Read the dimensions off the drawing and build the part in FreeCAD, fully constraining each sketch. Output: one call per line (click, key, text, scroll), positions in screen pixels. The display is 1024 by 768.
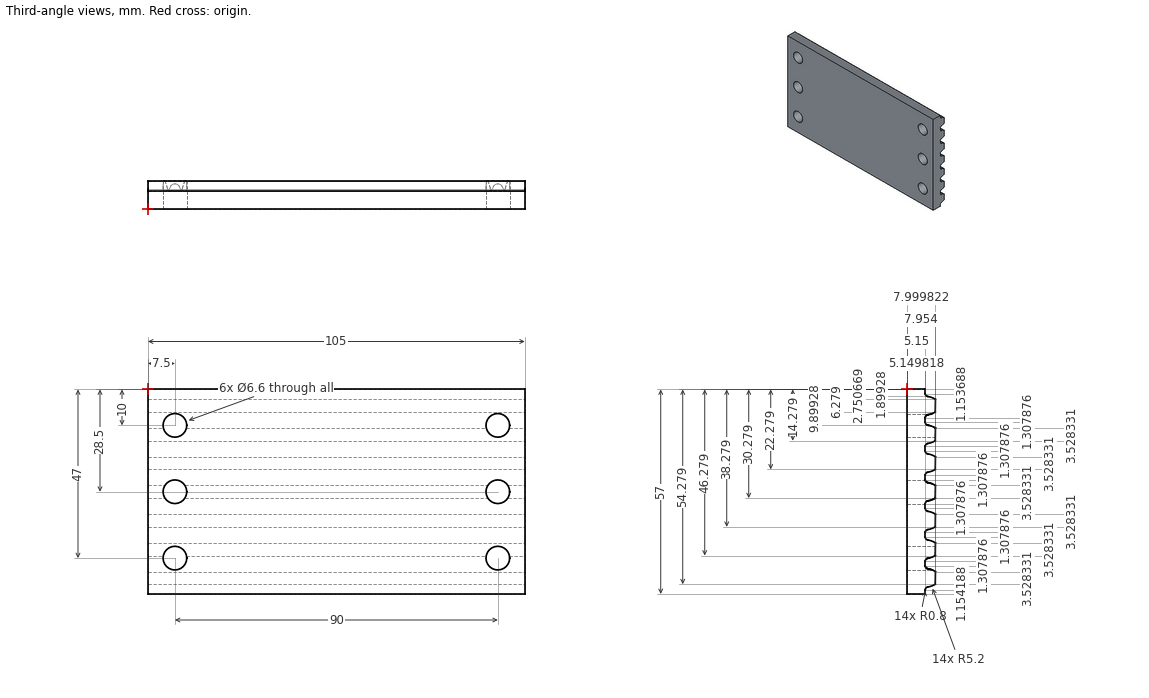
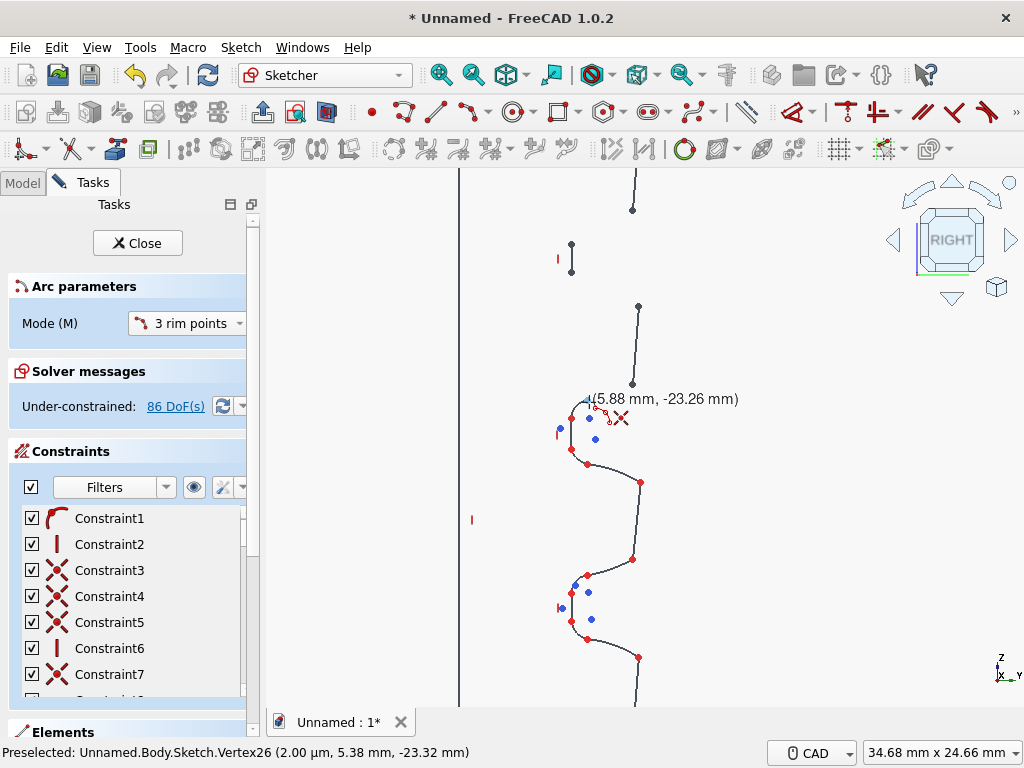
click(587, 401)
click(633, 385)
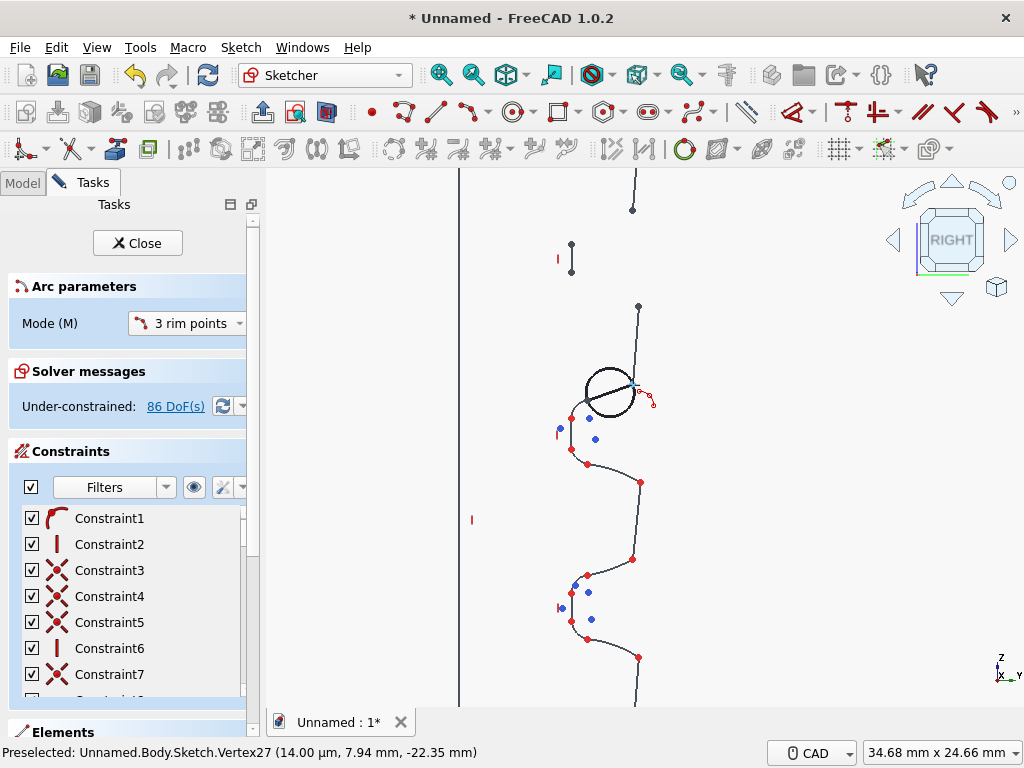
scroll(611, 394, up, 9)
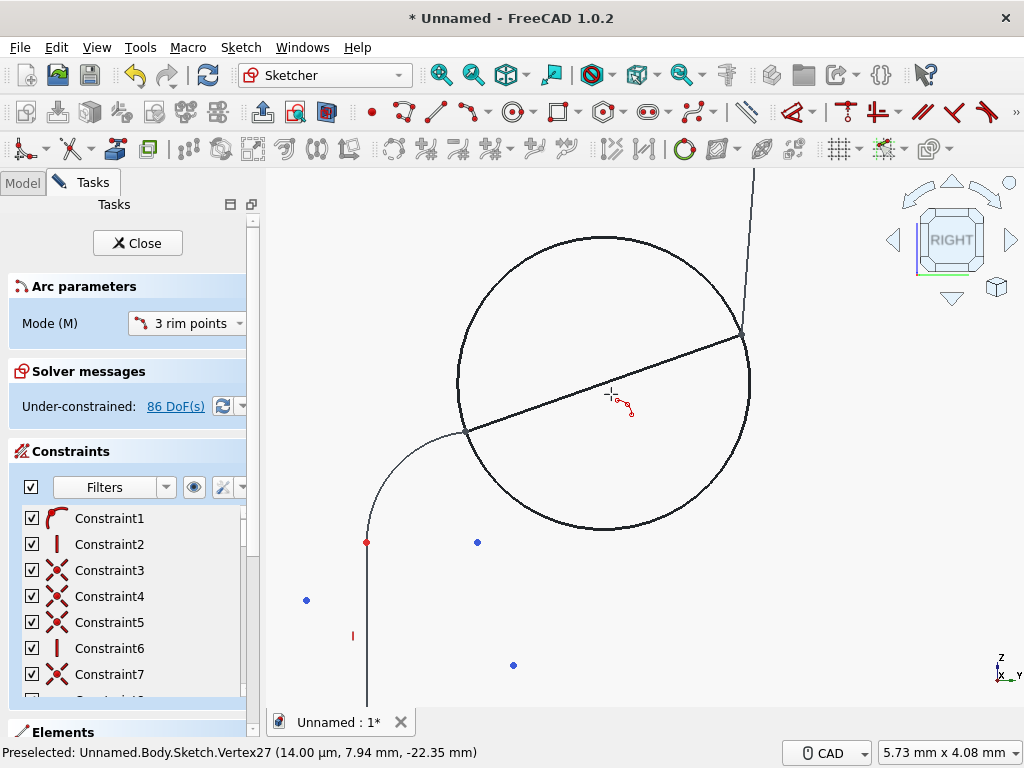
click(610, 391)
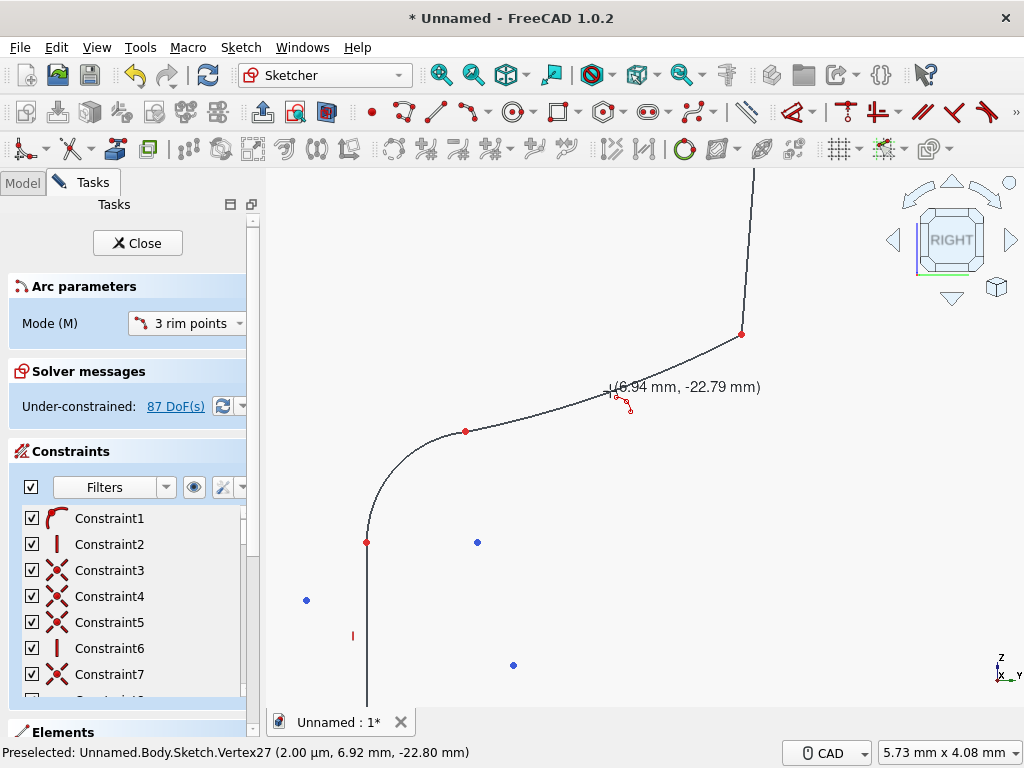
scroll(595, 400, down, 15)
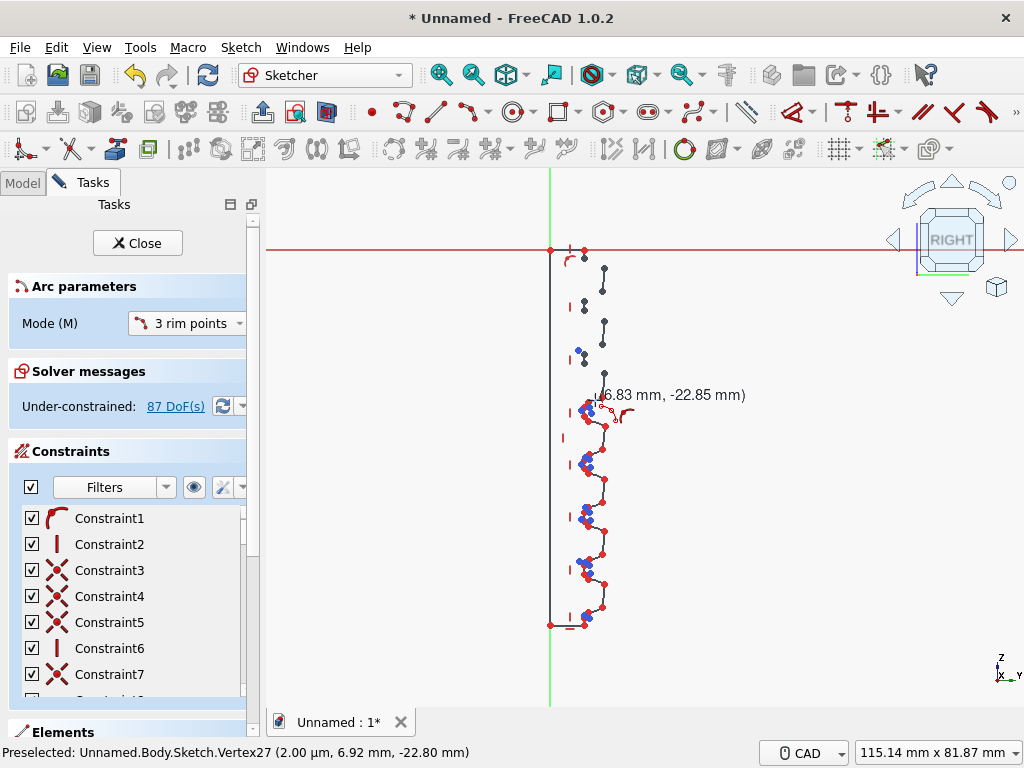
scroll(603, 373, up, 2)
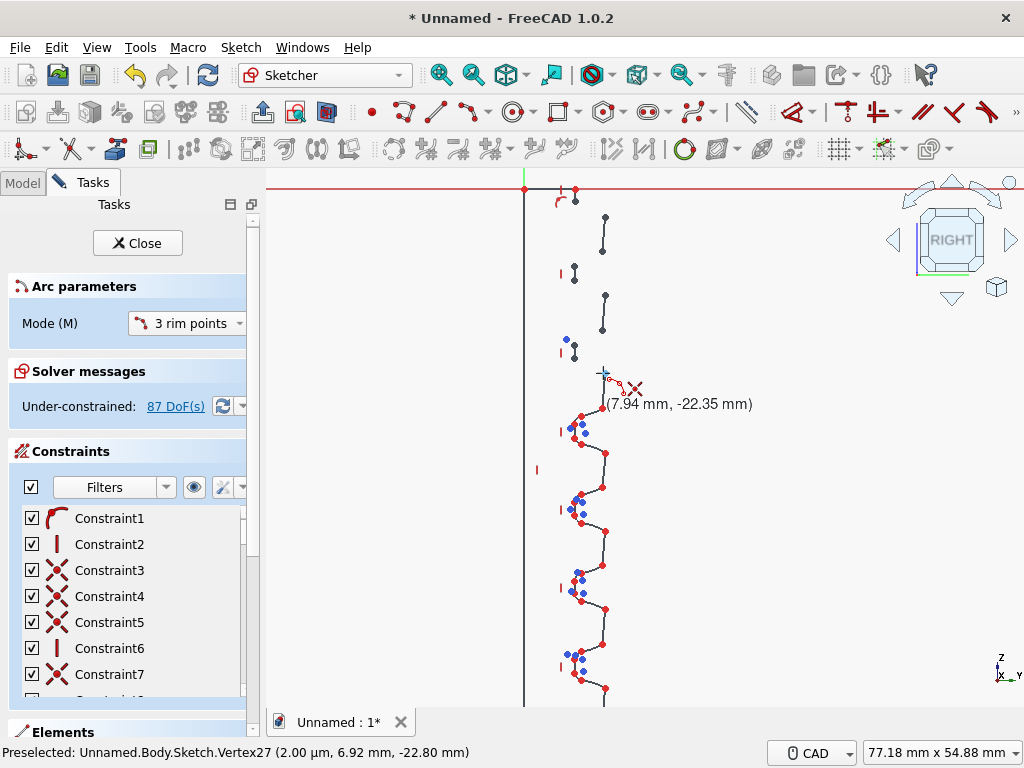
click(605, 374)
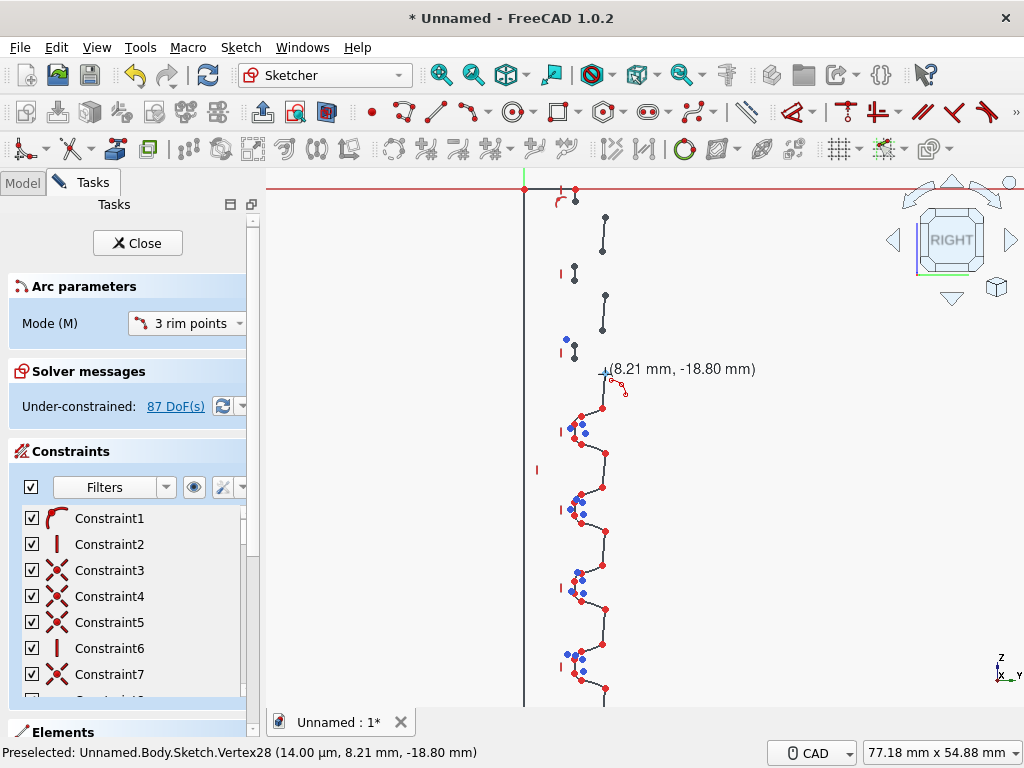
scroll(582, 366, up, 5)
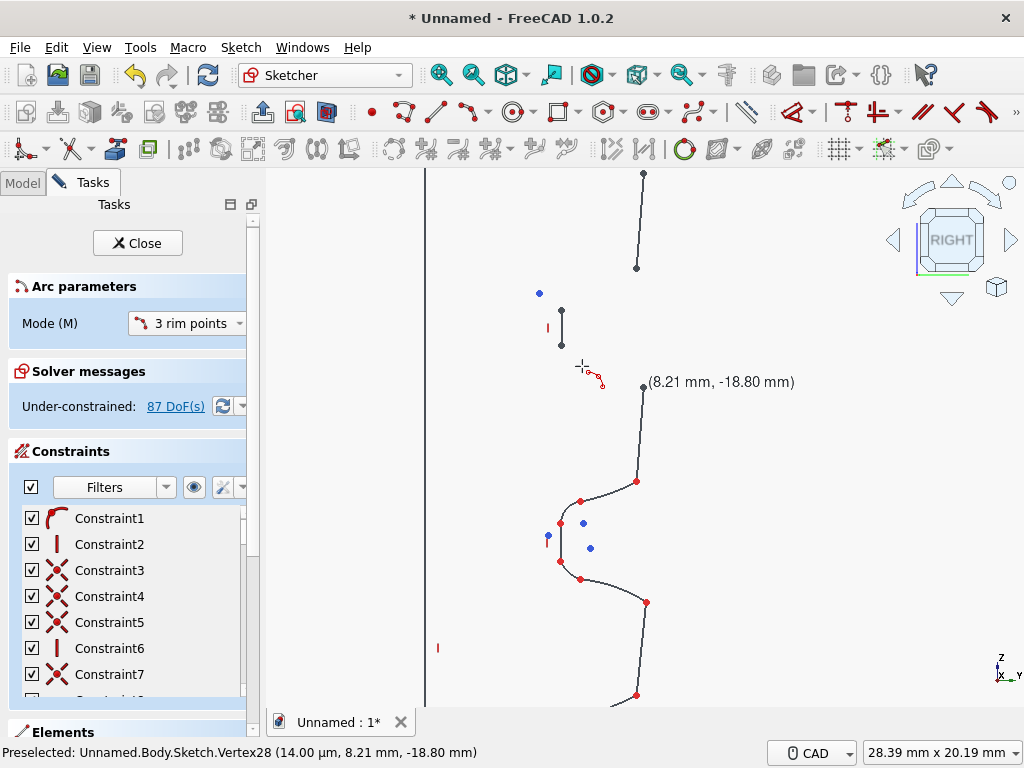
click(581, 364)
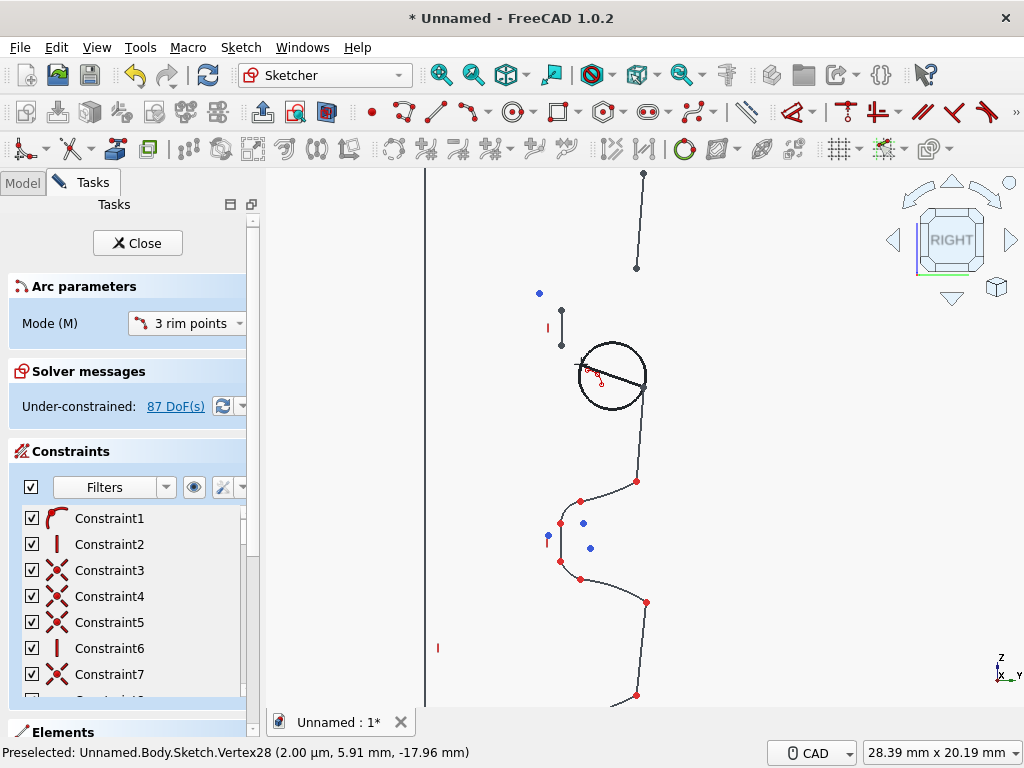
scroll(611, 372, up, 8)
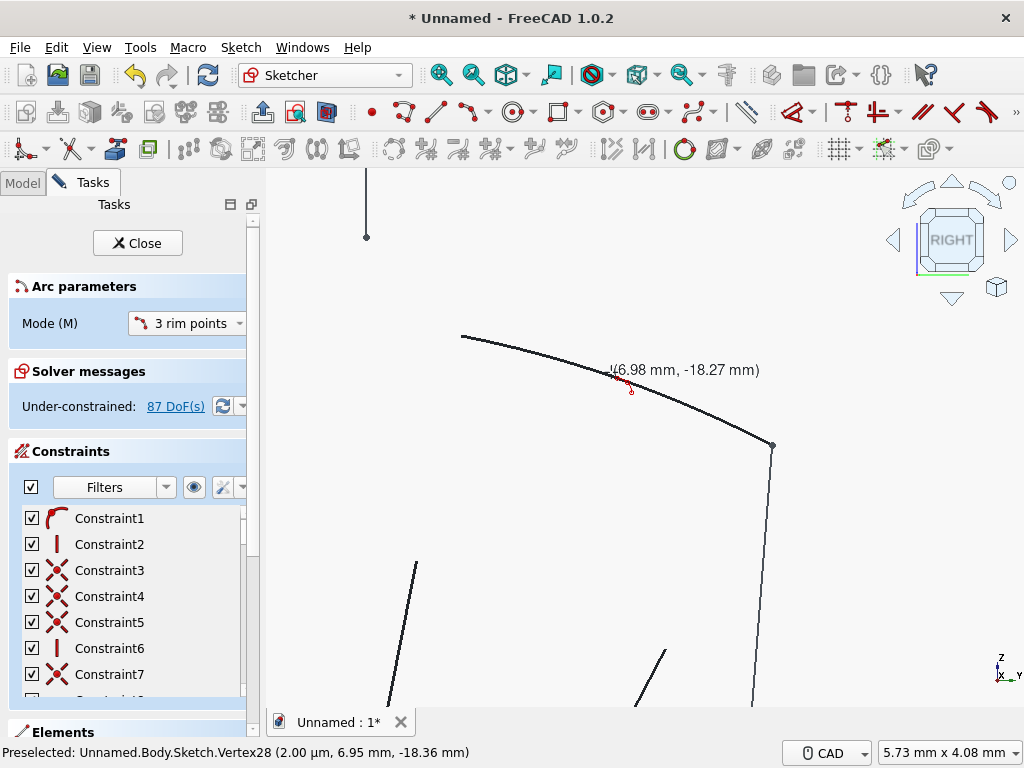
click(608, 369)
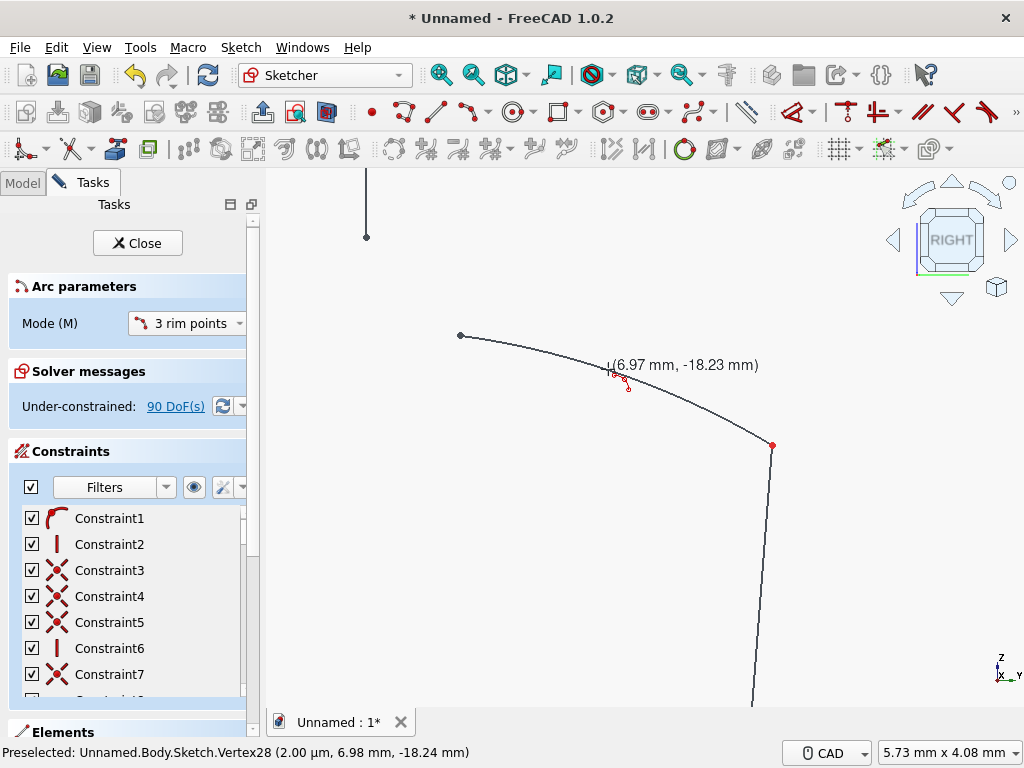
scroll(595, 370, down, 15)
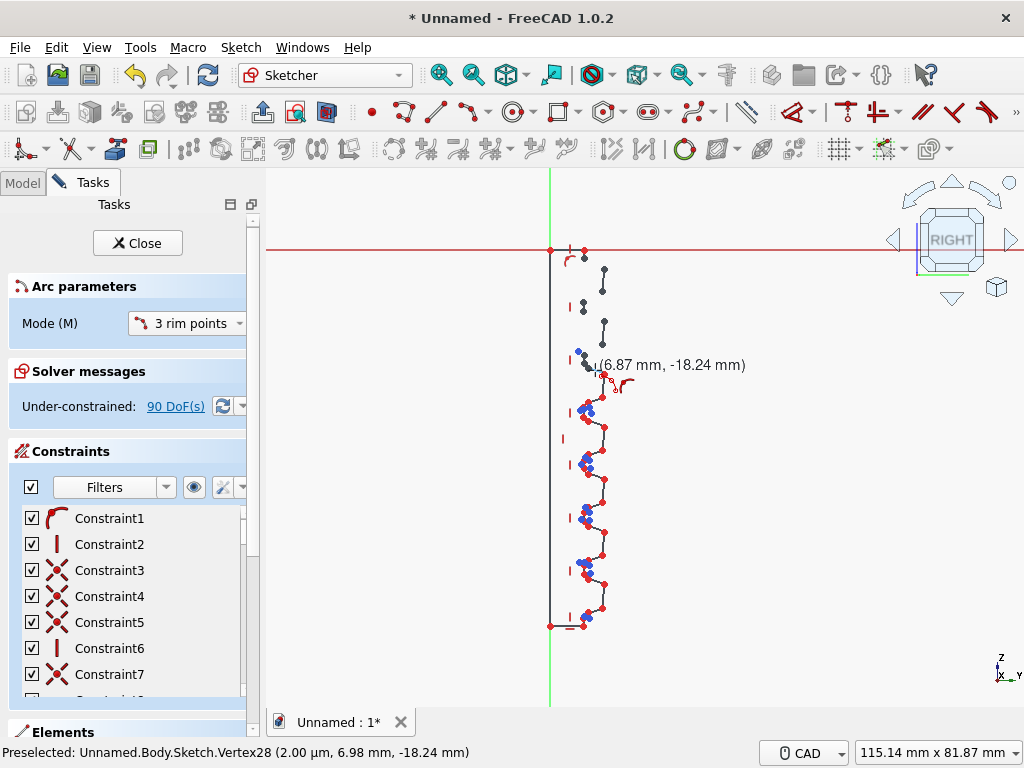
scroll(589, 368, up, 7)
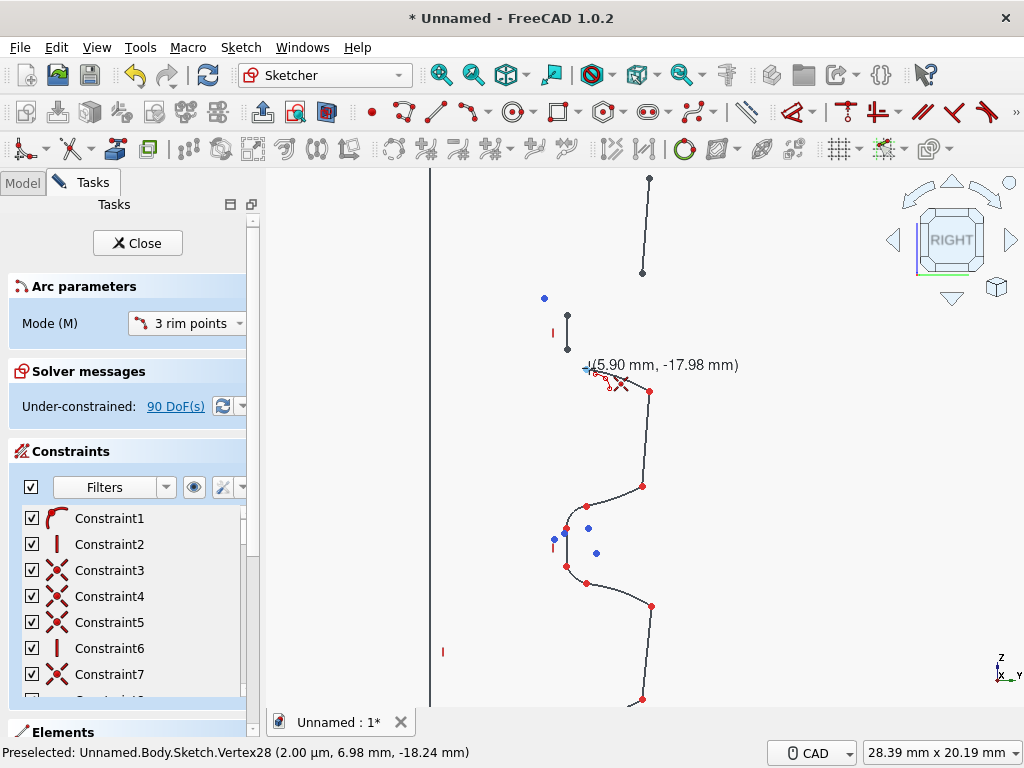
click(587, 370)
click(567, 350)